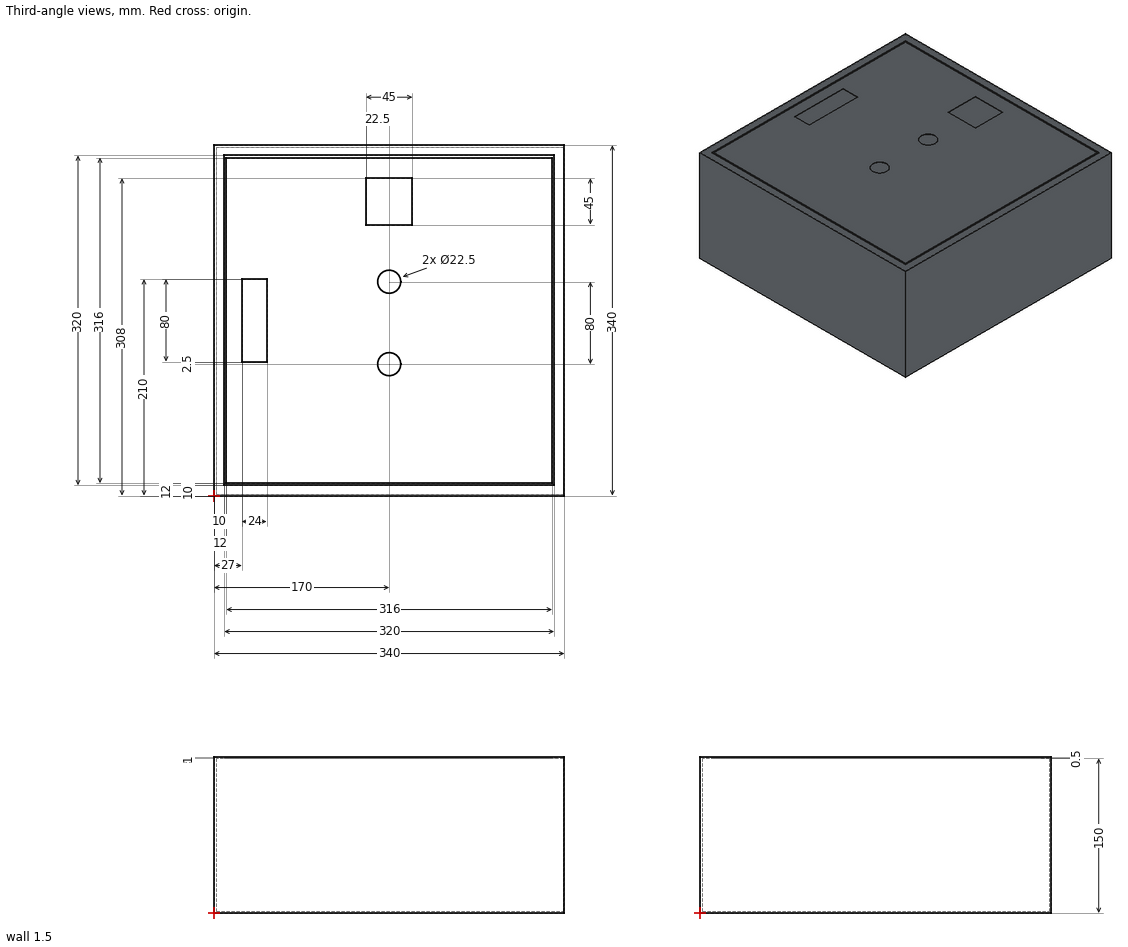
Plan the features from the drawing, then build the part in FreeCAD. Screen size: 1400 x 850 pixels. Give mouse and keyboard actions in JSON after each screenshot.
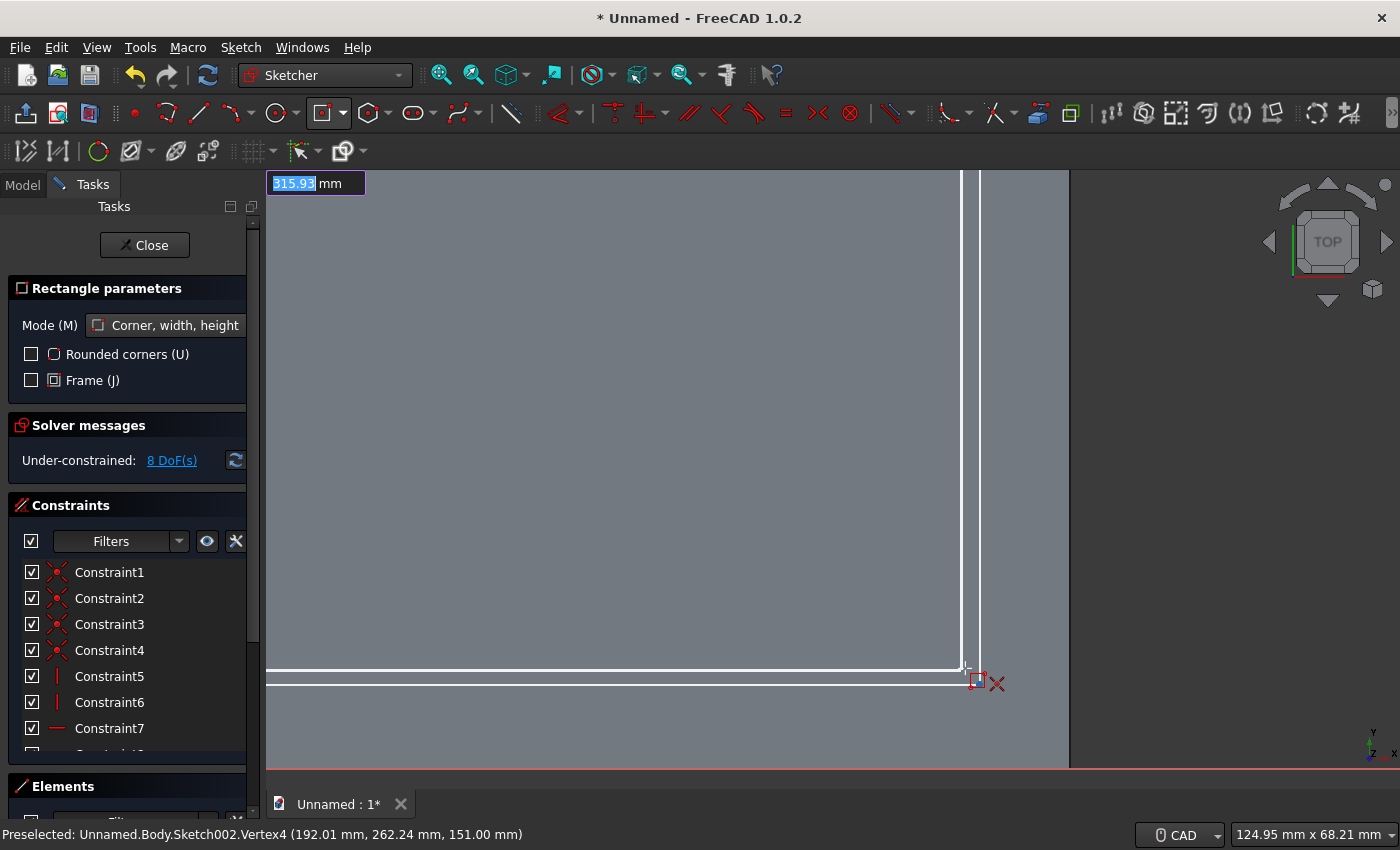
{"action": "left_click", "coordinate": [961, 660]}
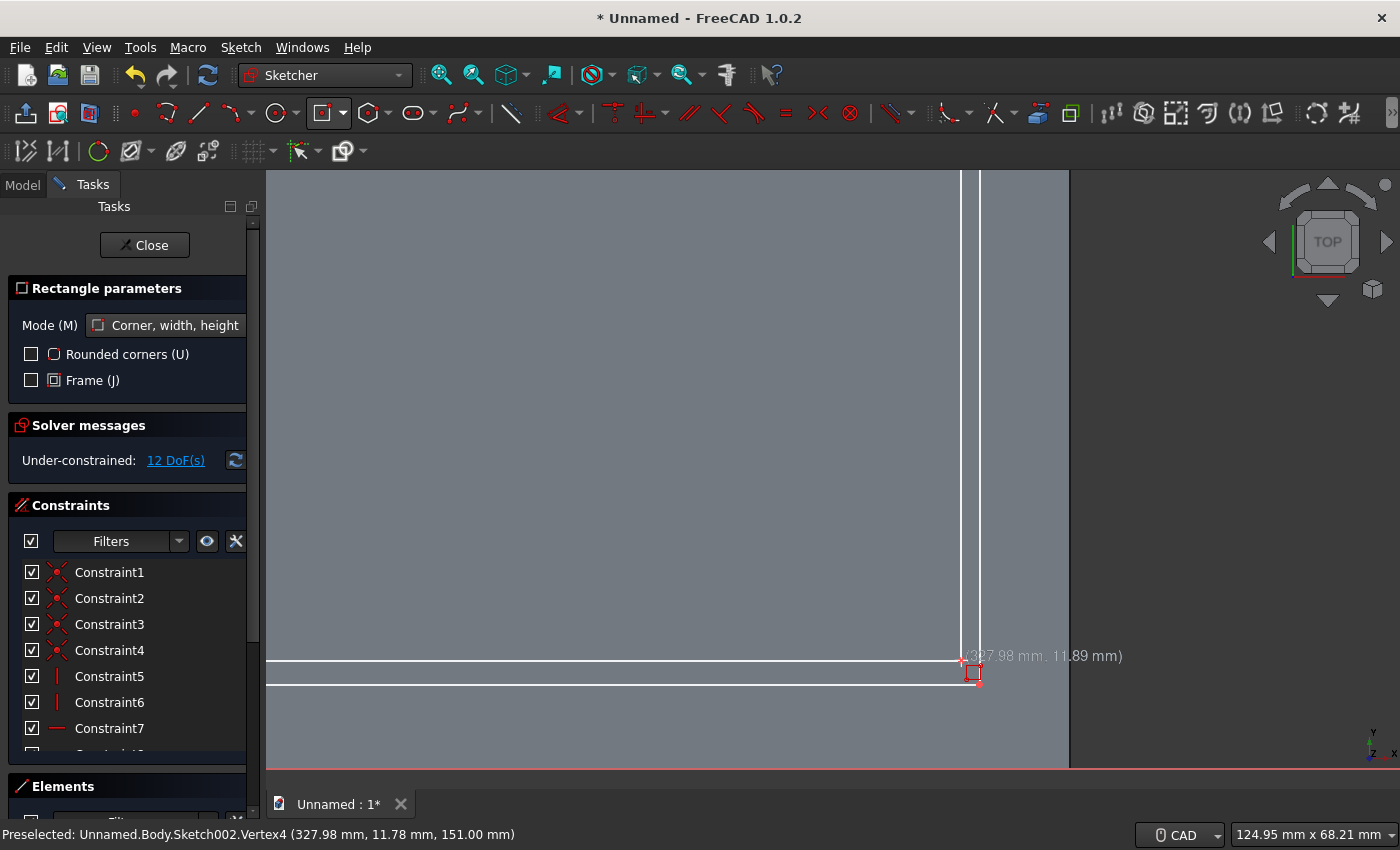
{"action": "left_click", "coordinate": [276, 114]}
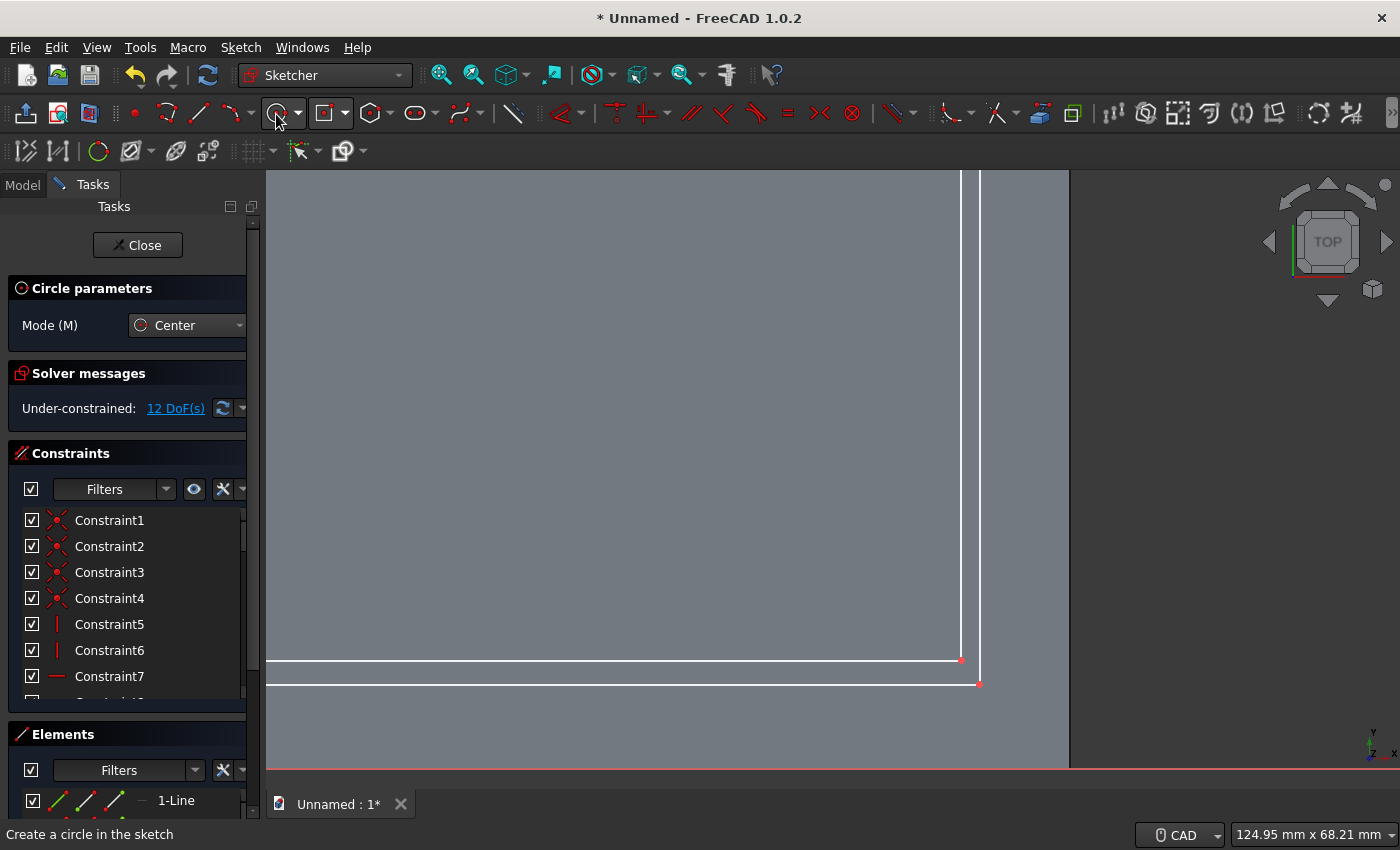
{"action": "scroll", "coordinate": [965, 669], "scroll_direction": "down", "scroll_amount": 10}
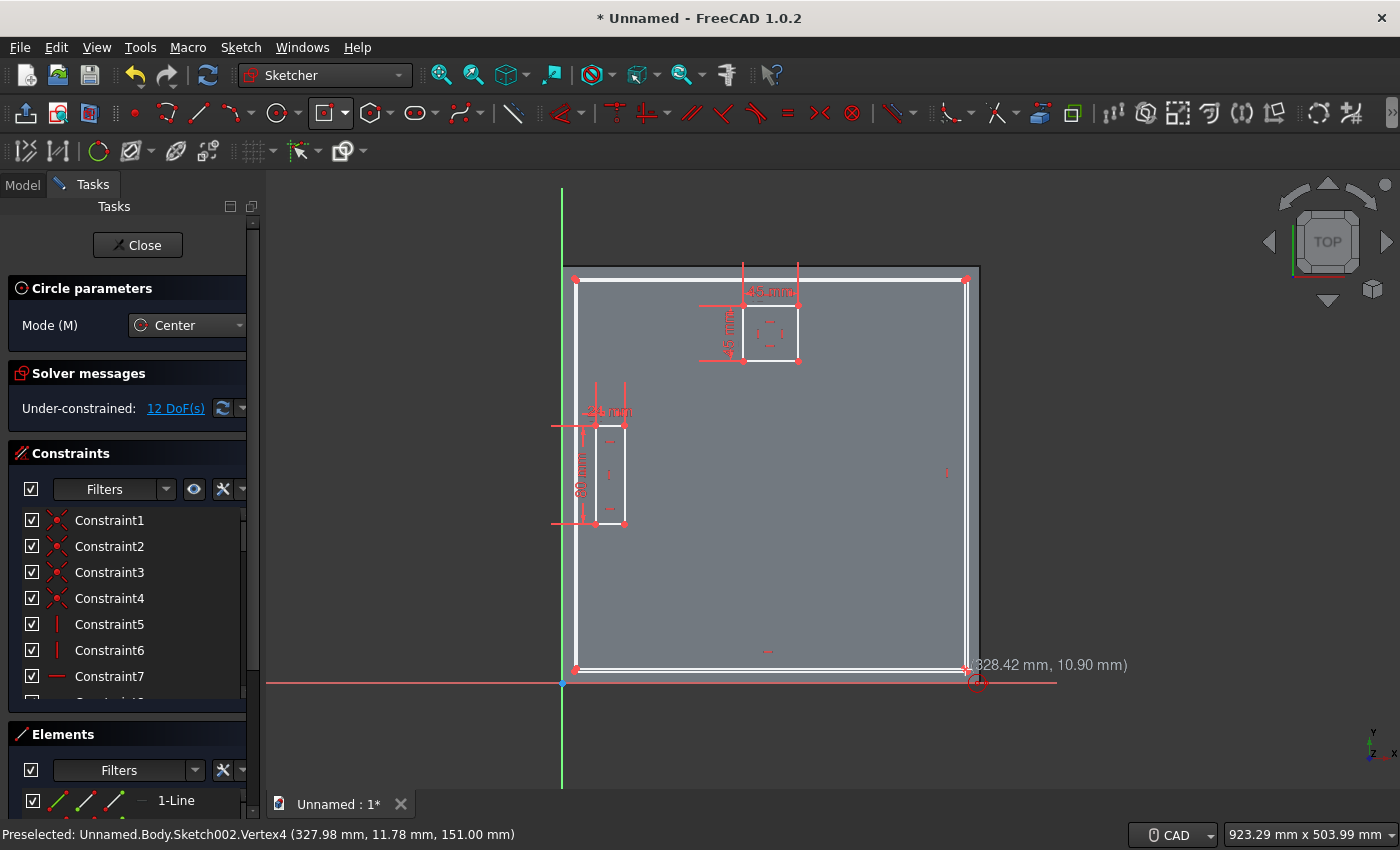
{"action": "scroll", "coordinate": [771, 428], "scroll_direction": "up", "scroll_amount": 3}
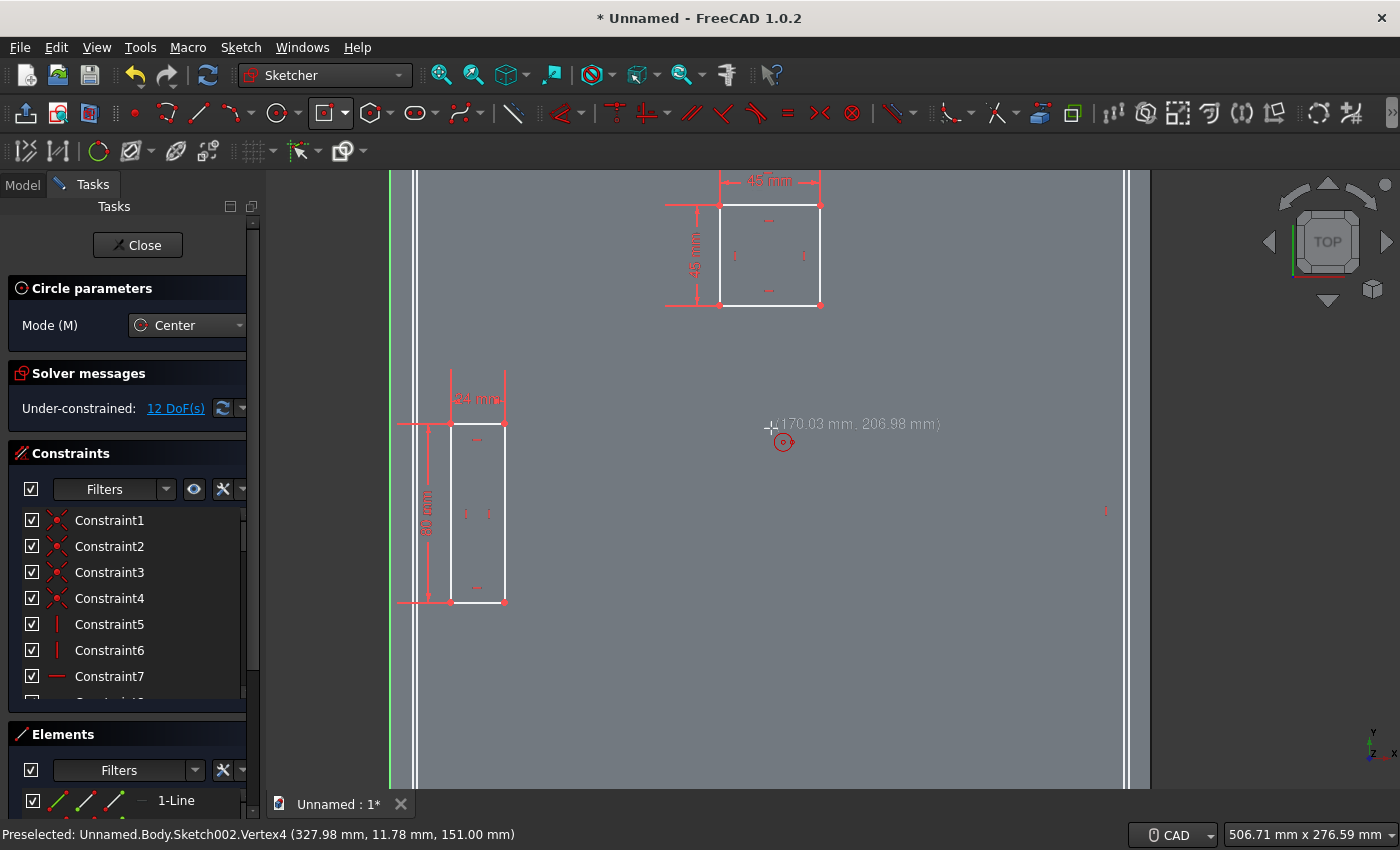
{"action": "left_click", "coordinate": [771, 428]}
{"action": "mouse_move", "coordinate": [788, 411]}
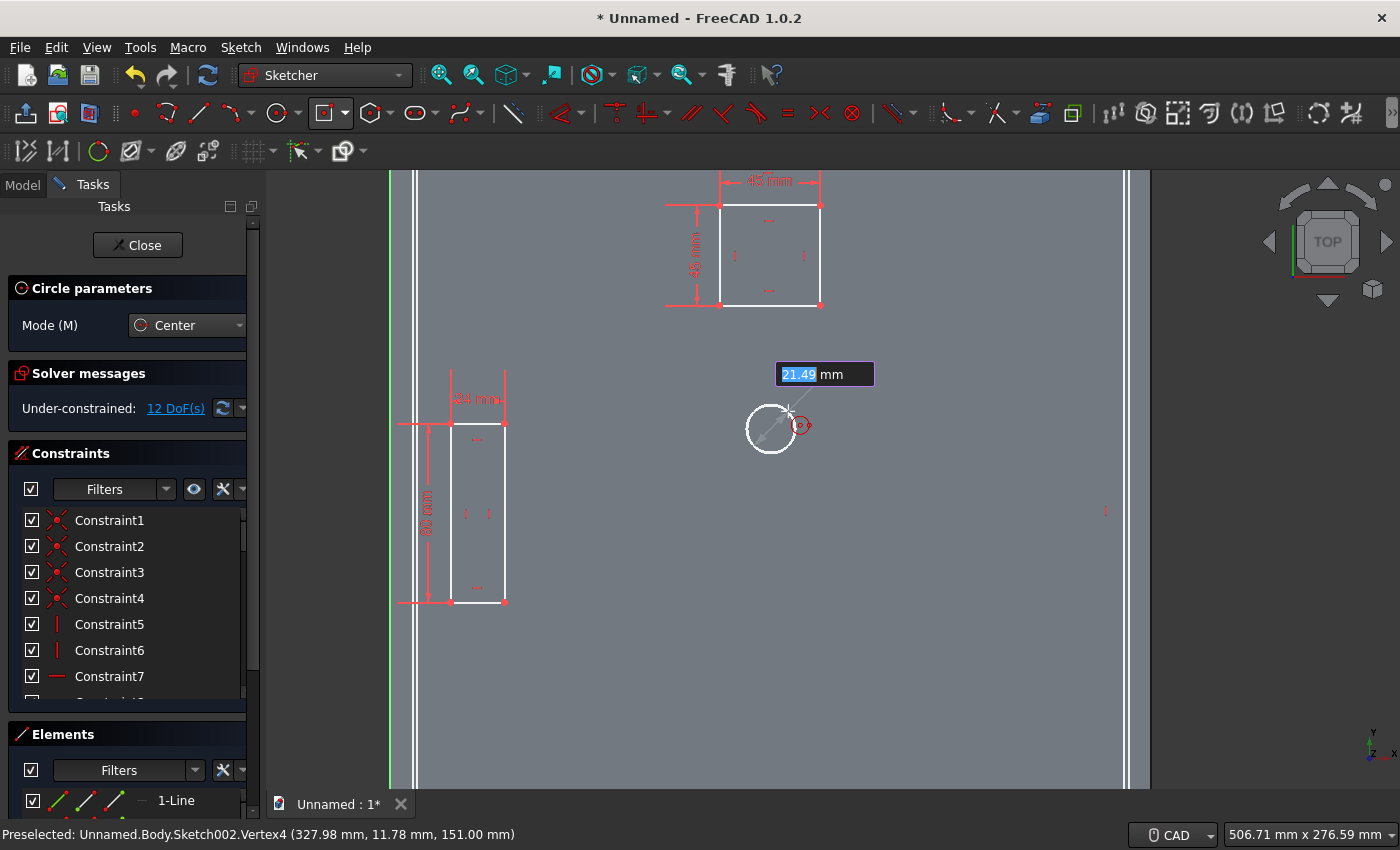
{"action": "type", "text": "22.5"}
{"action": "key", "text": "Return"}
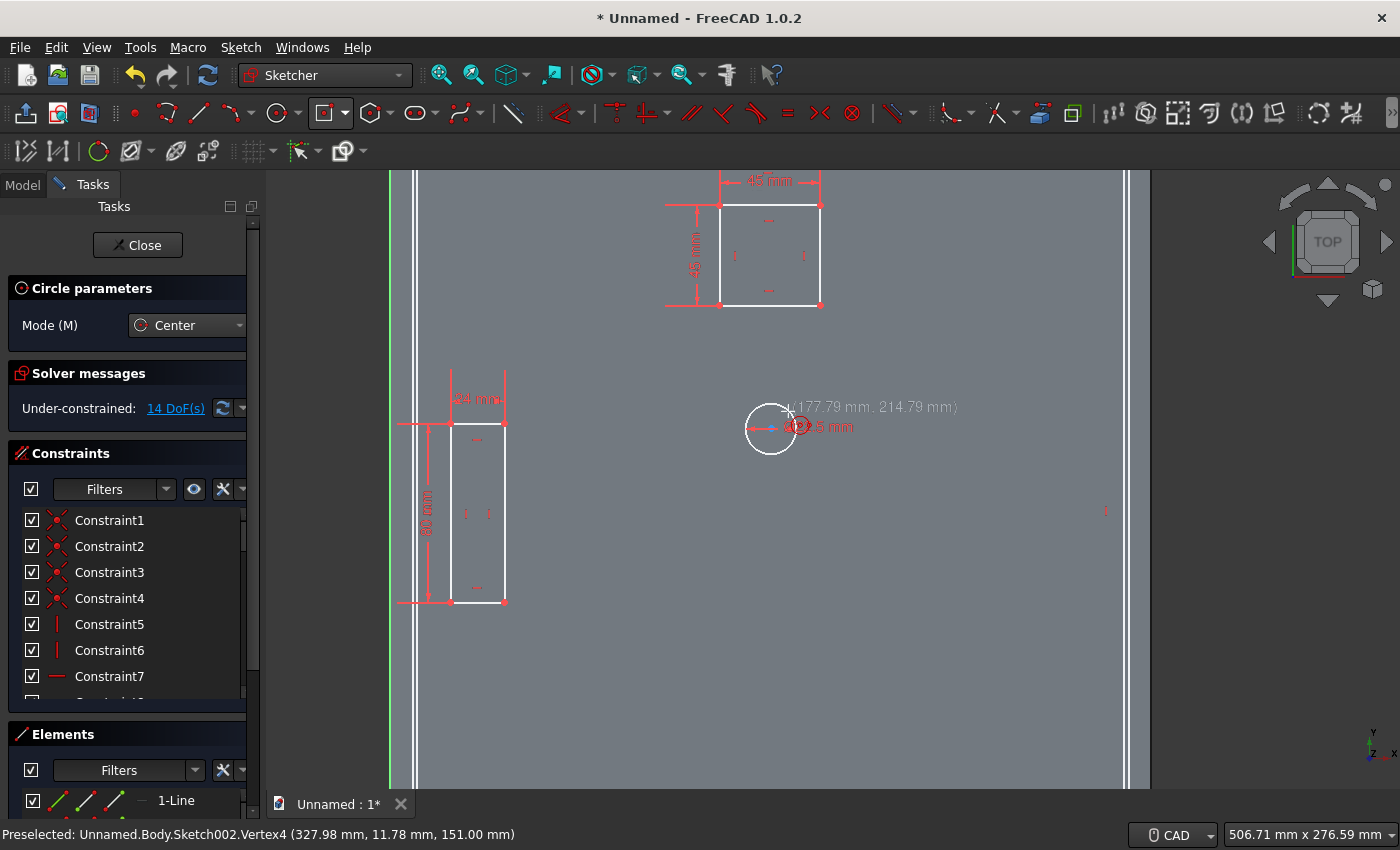
{"action": "left_click", "coordinate": [771, 607]}
{"action": "mouse_move", "coordinate": [788, 590]}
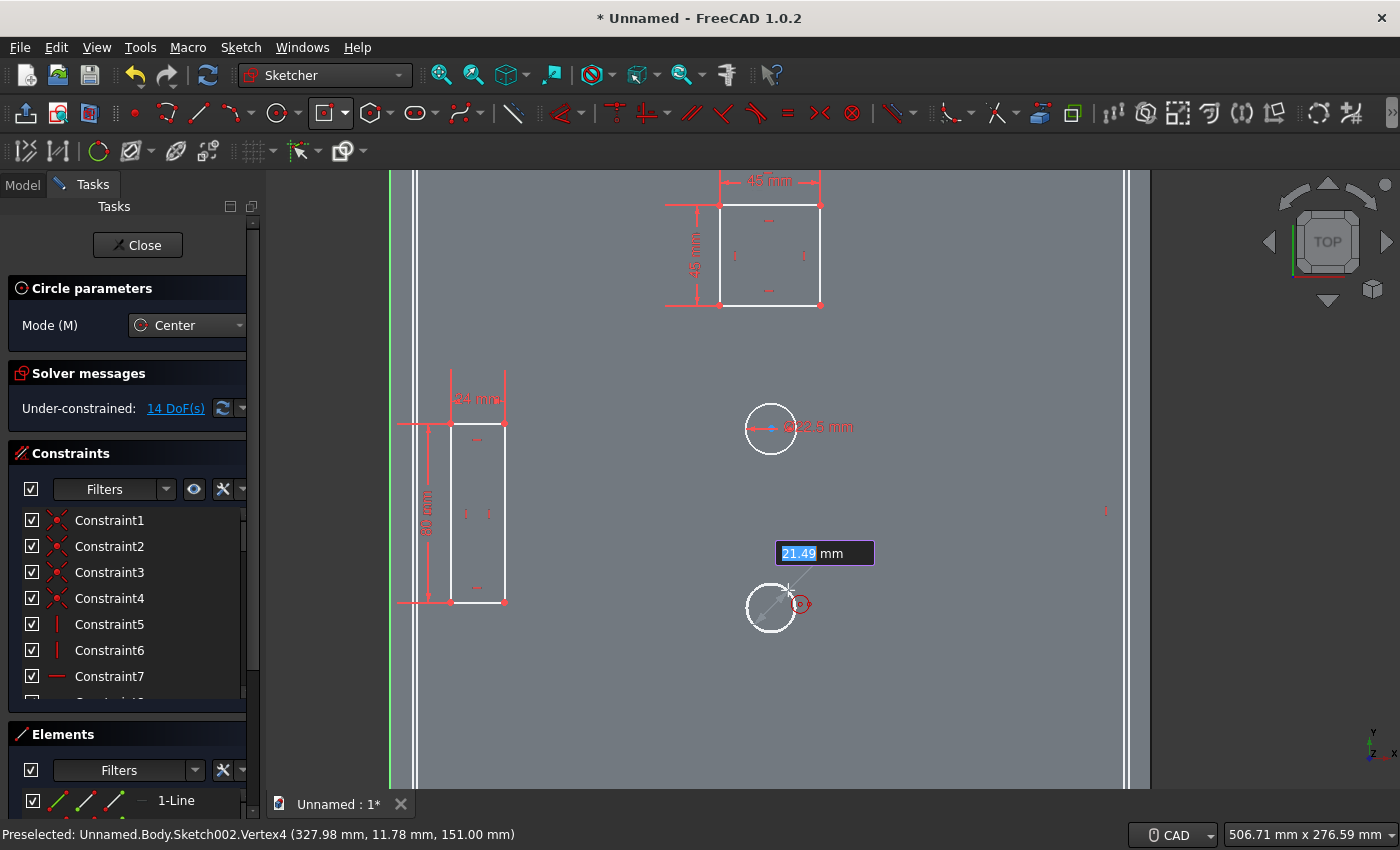
{"action": "type", "text": "22.5"}
{"action": "key", "text": "Return"}
{"action": "key", "text": "Escape"}